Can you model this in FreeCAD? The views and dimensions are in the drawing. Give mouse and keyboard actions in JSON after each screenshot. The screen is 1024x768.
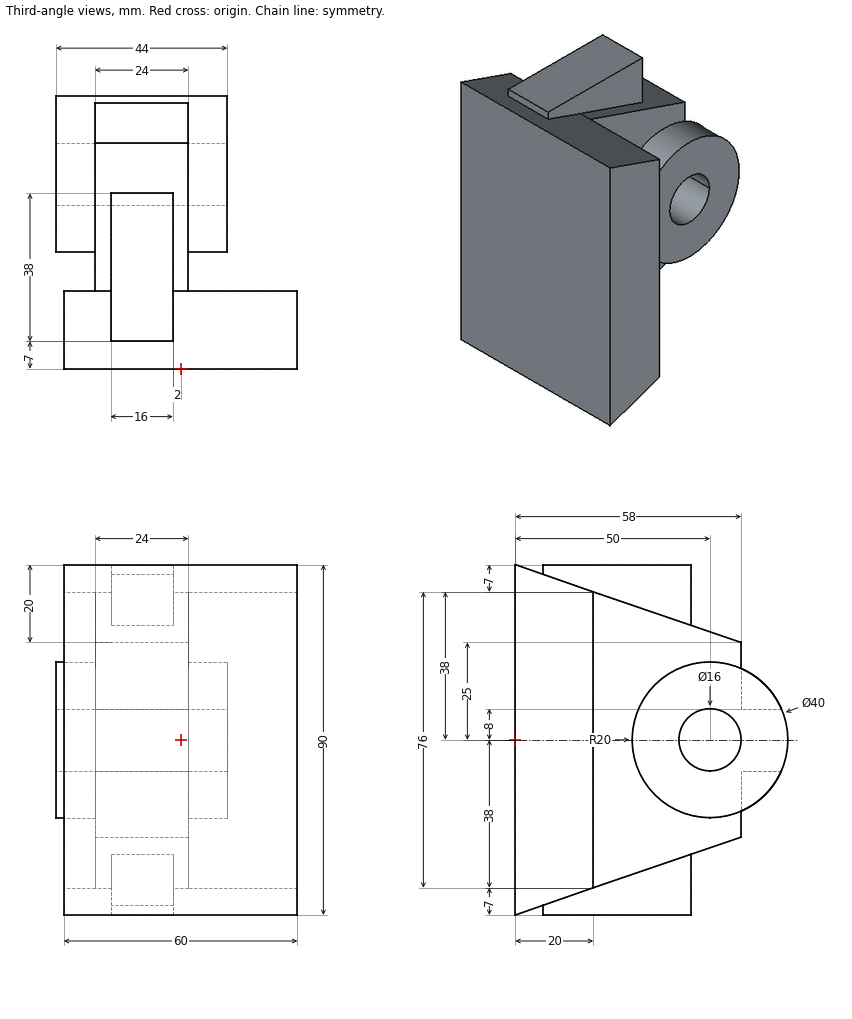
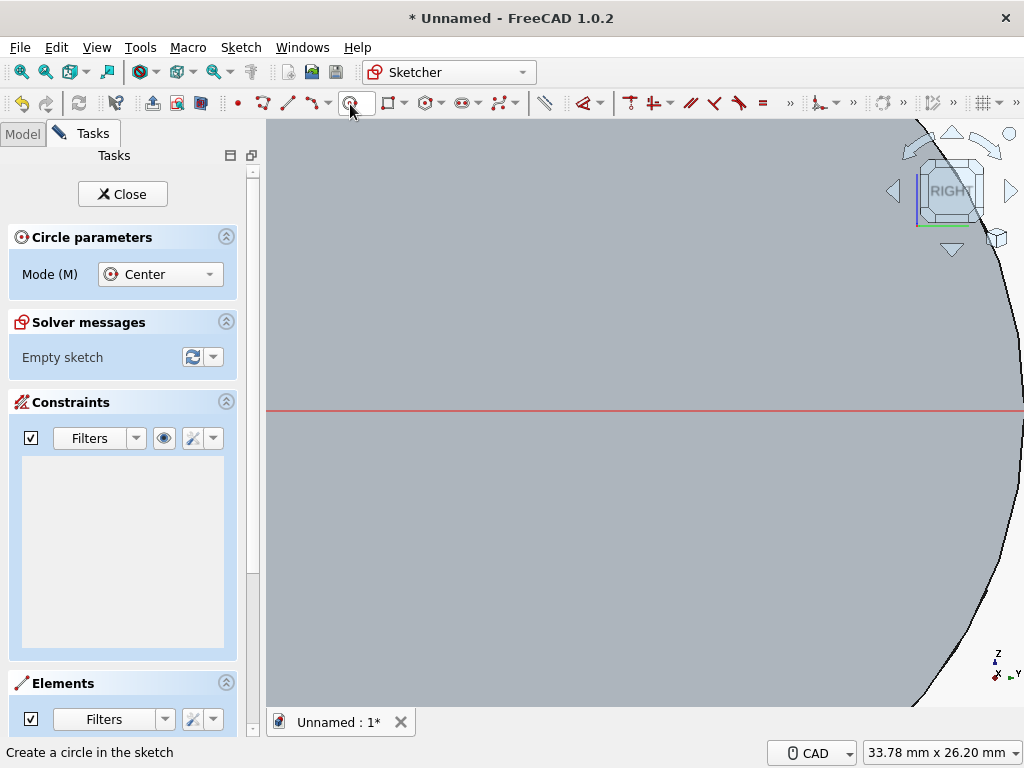
{"action": "left_click", "coordinate": [576, 411]}
{"action": "mouse_move", "coordinate": [703, 284]}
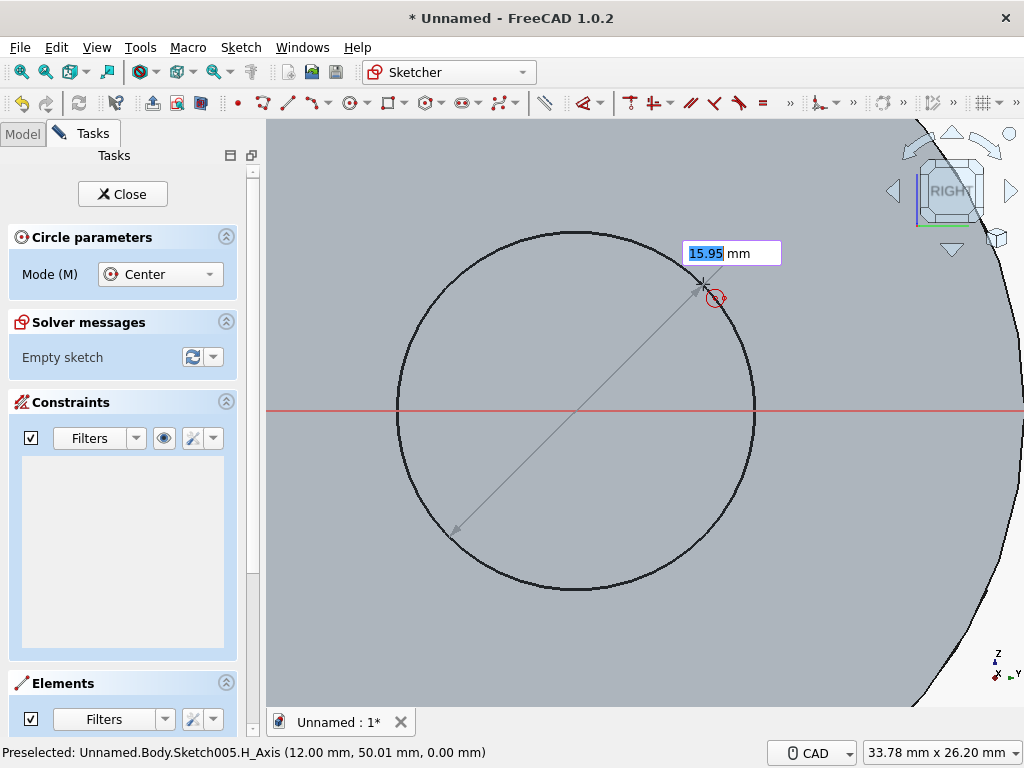
{"action": "type", "text": "16"}
{"action": "key", "text": "Return"}
{"action": "key", "text": "Escape"}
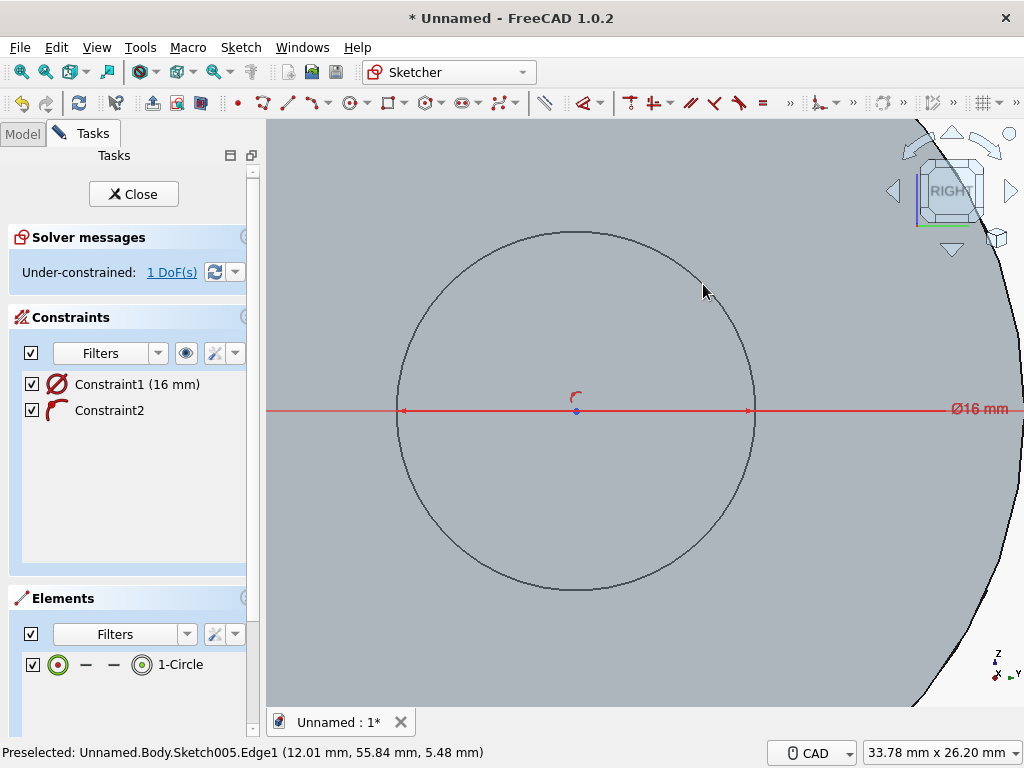
{"action": "left_click", "coordinate": [584, 104]}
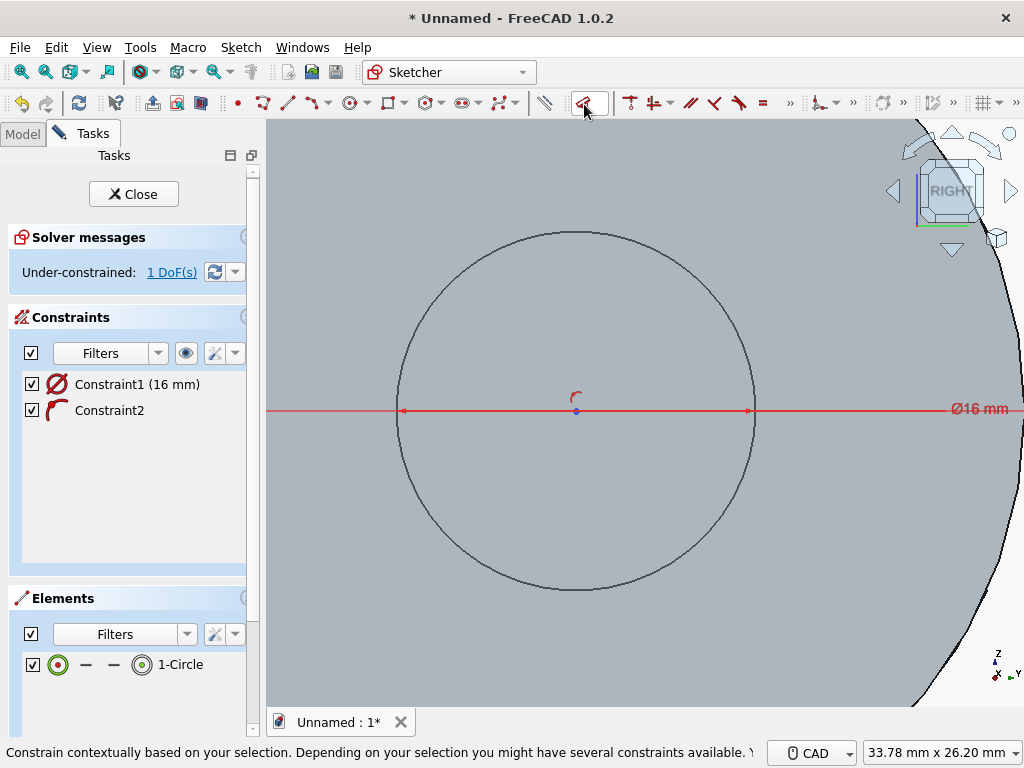
{"action": "left_click", "coordinate": [576, 411]}
{"action": "left_click", "coordinate": [435, 445]}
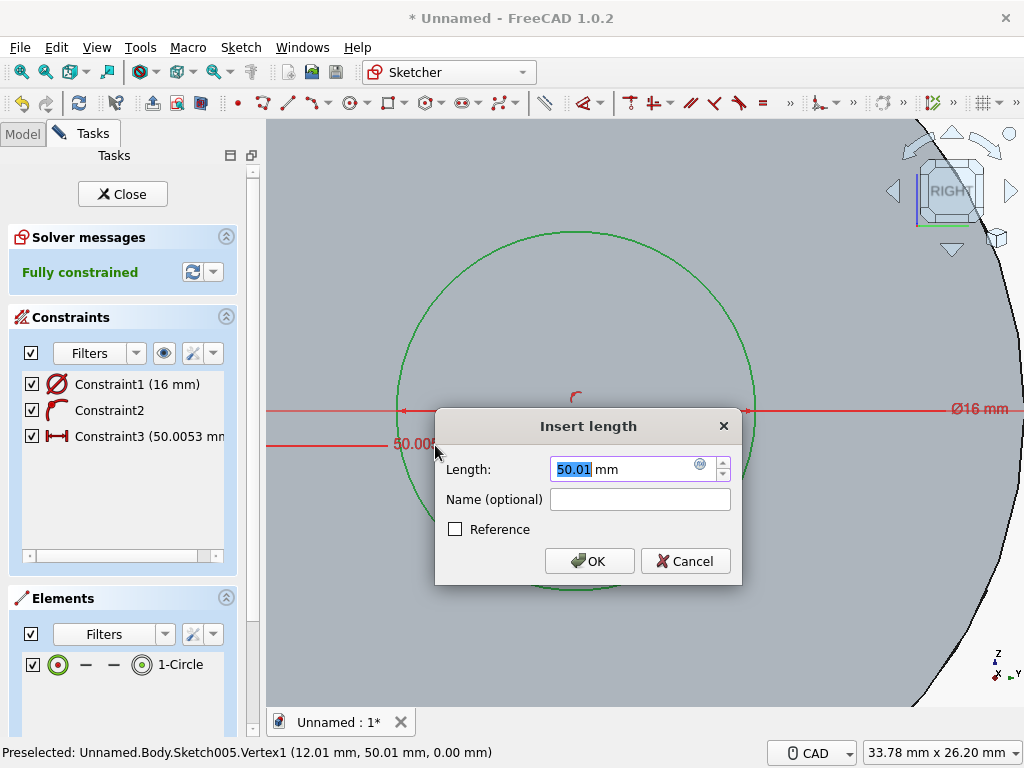
{"action": "type", "text": "50"}
{"action": "key", "text": "Return"}
{"action": "key", "text": "Escape"}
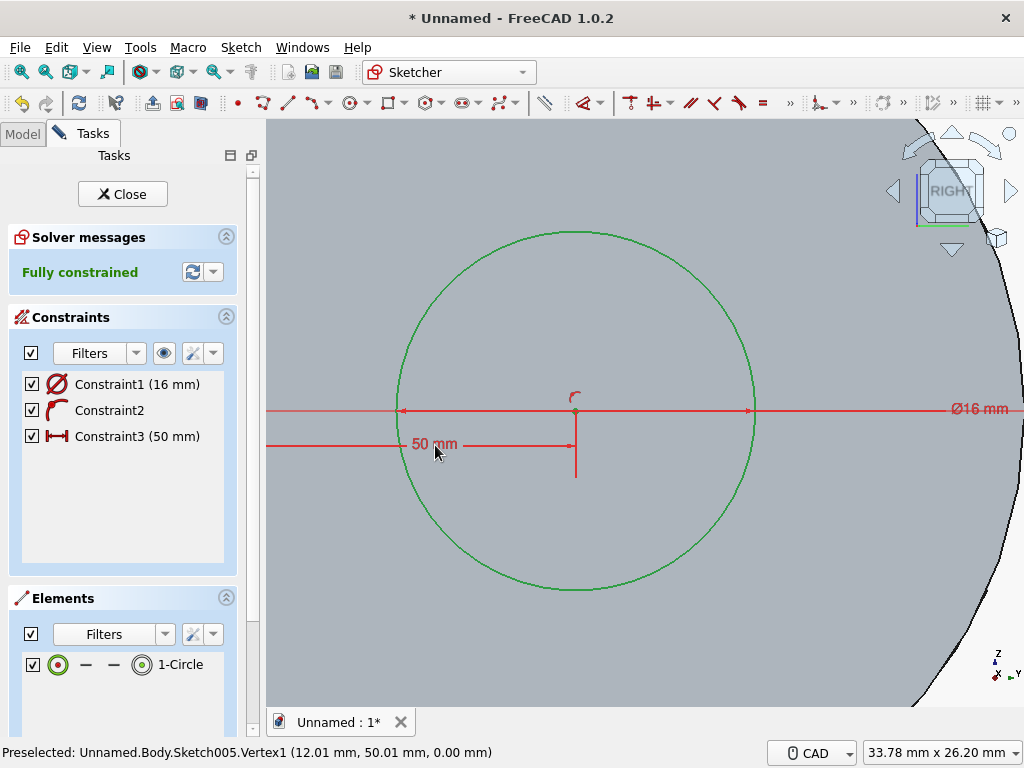
{"action": "left_click", "coordinate": [123, 194]}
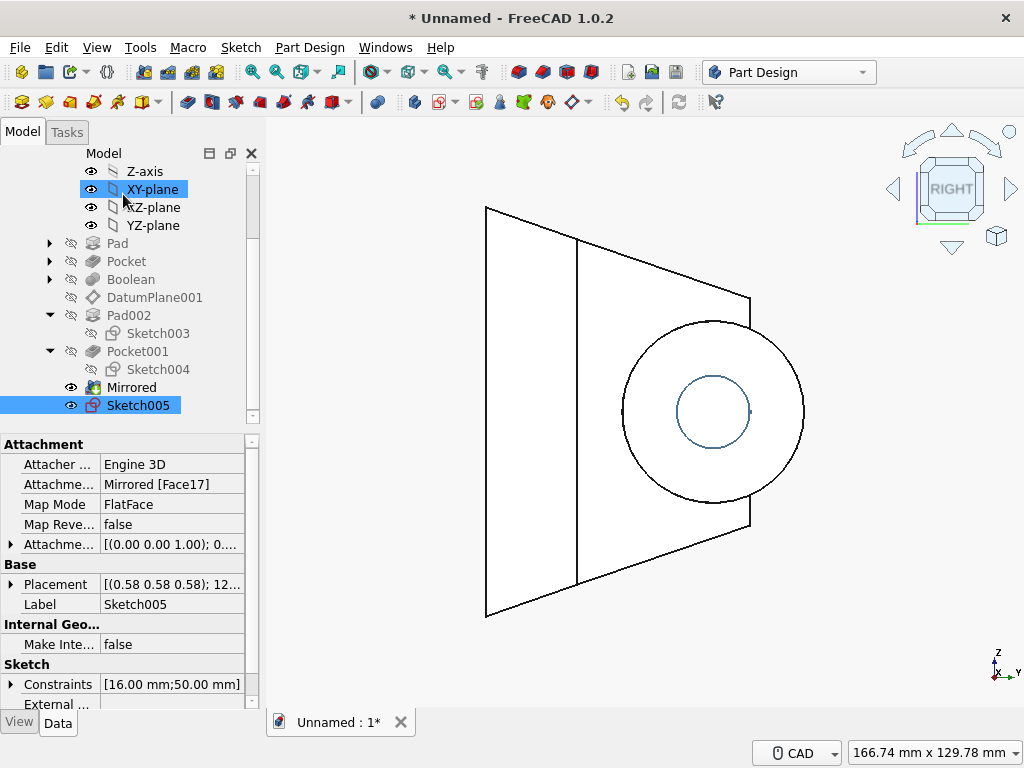
{"action": "left_click", "coordinate": [188, 102]}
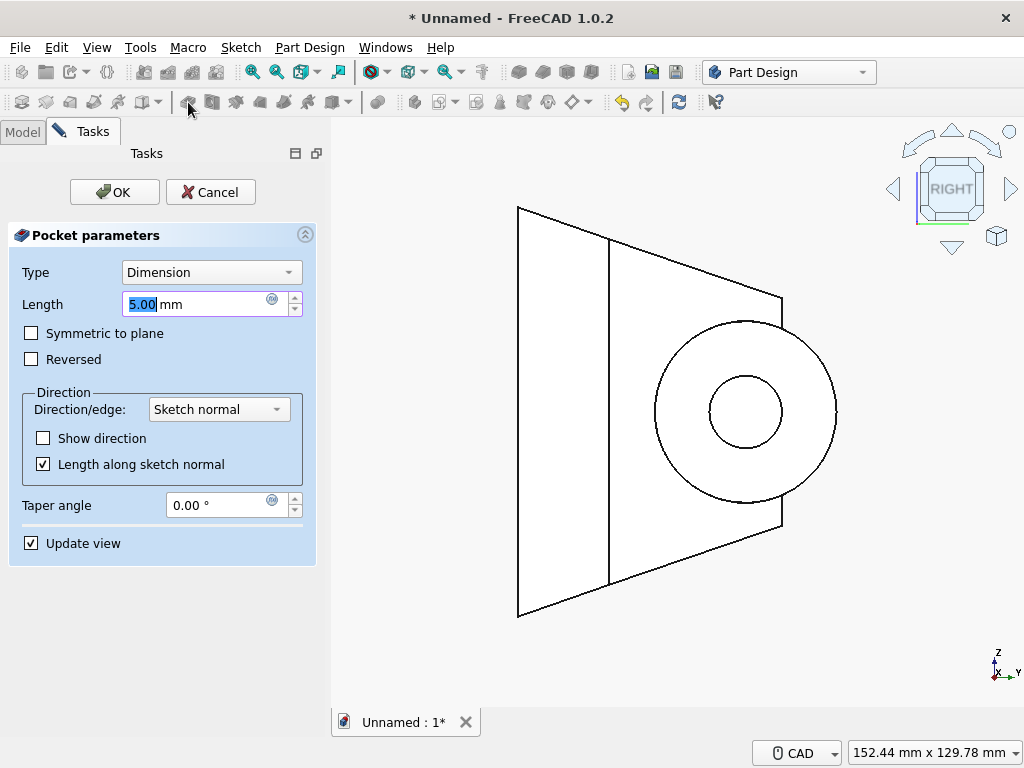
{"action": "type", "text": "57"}
{"action": "key", "text": "Tab"}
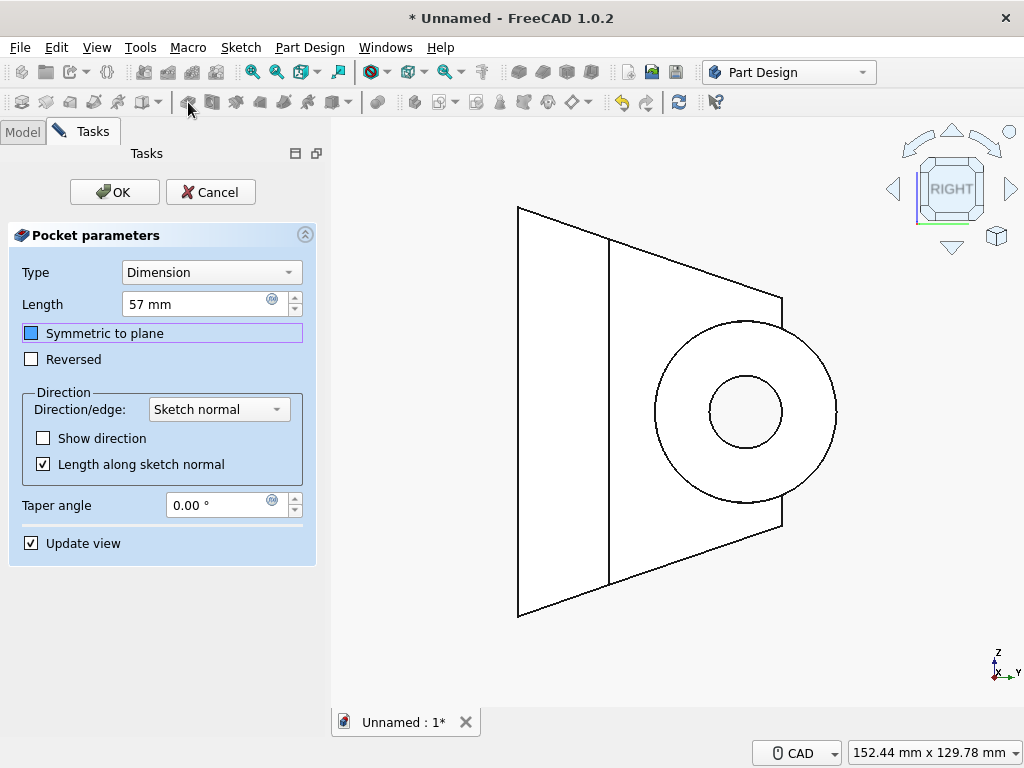
{"action": "left_click", "coordinate": [115, 192]}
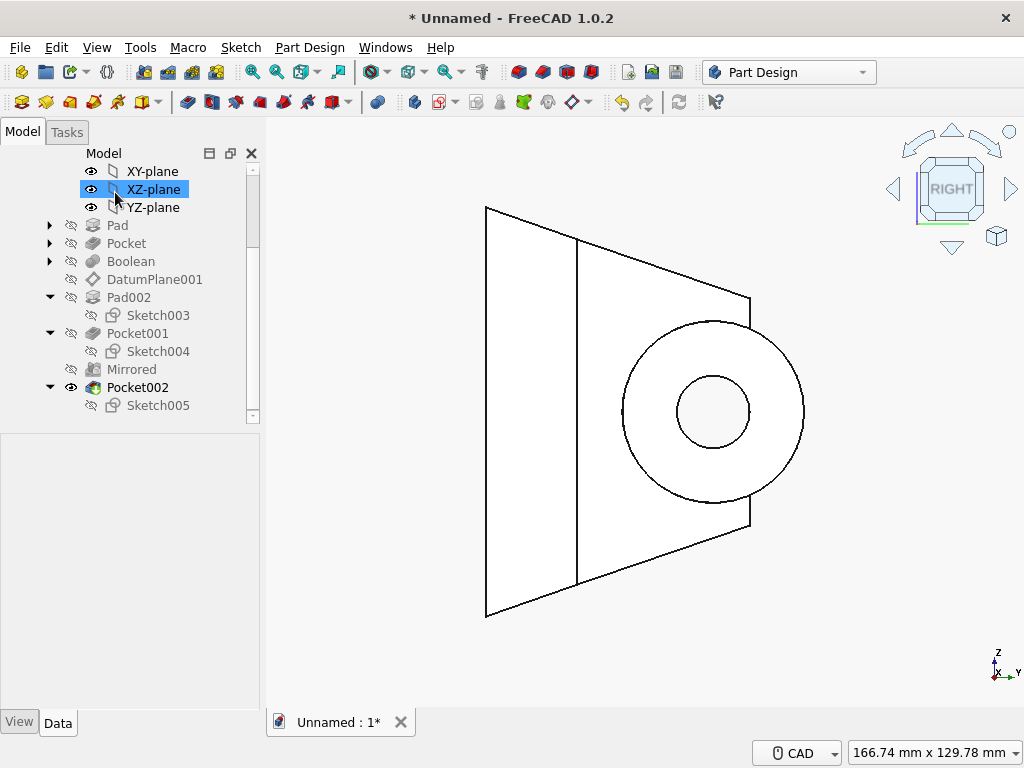
{"action": "scroll", "coordinate": [160, 293], "scroll_direction": "down", "scroll_amount": 3}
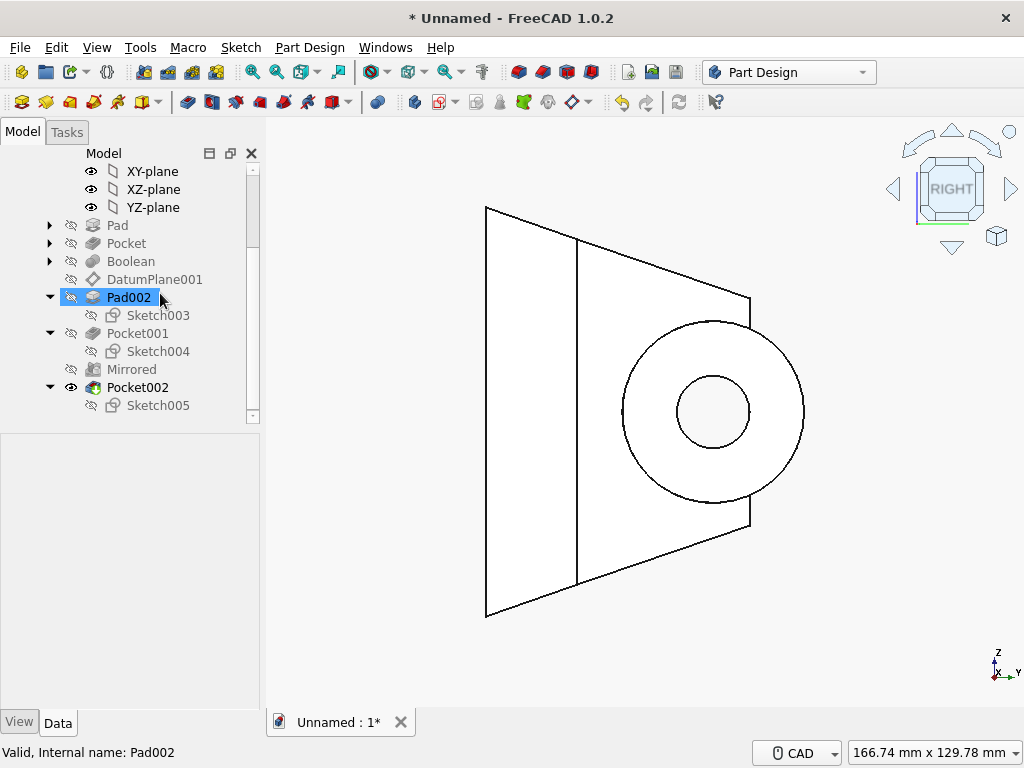
{"action": "scroll", "coordinate": [160, 293], "scroll_direction": "up", "scroll_amount": 15}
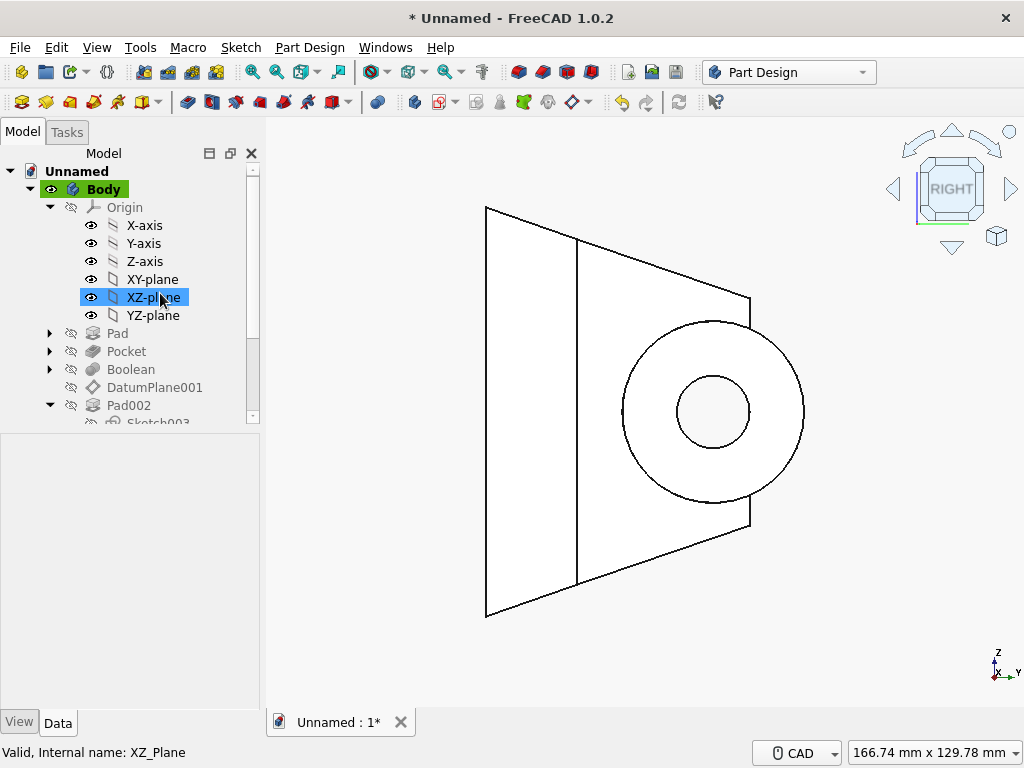
{"action": "left_click", "coordinate": [136, 279]}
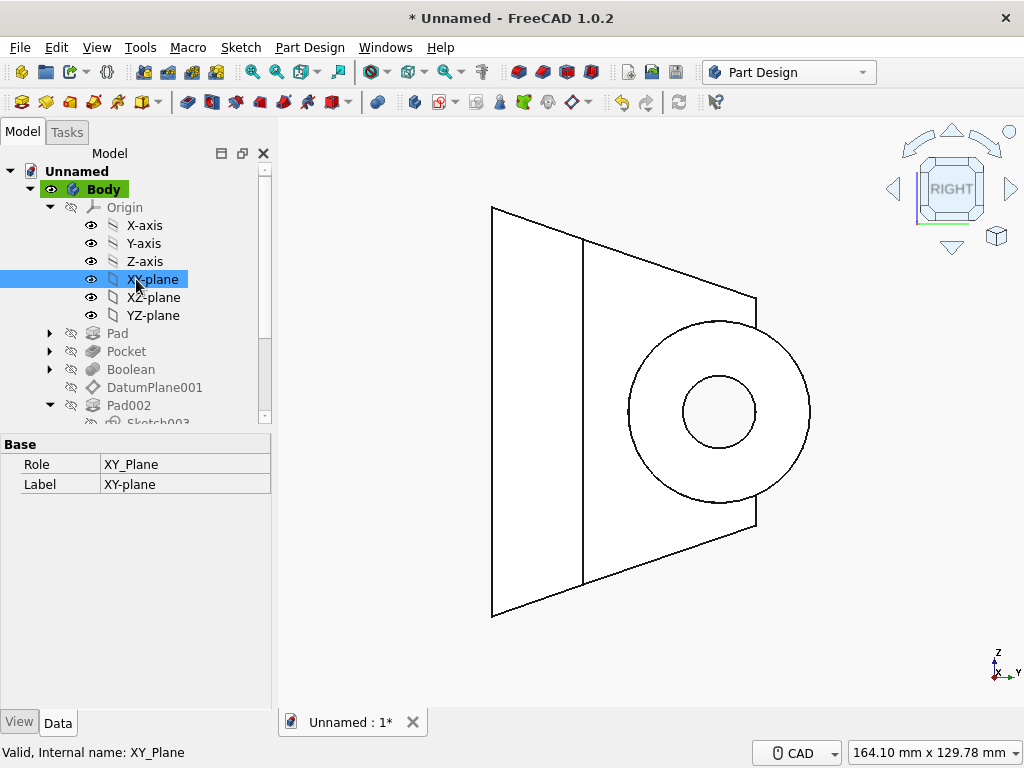
{"action": "left_click", "coordinate": [572, 102]}